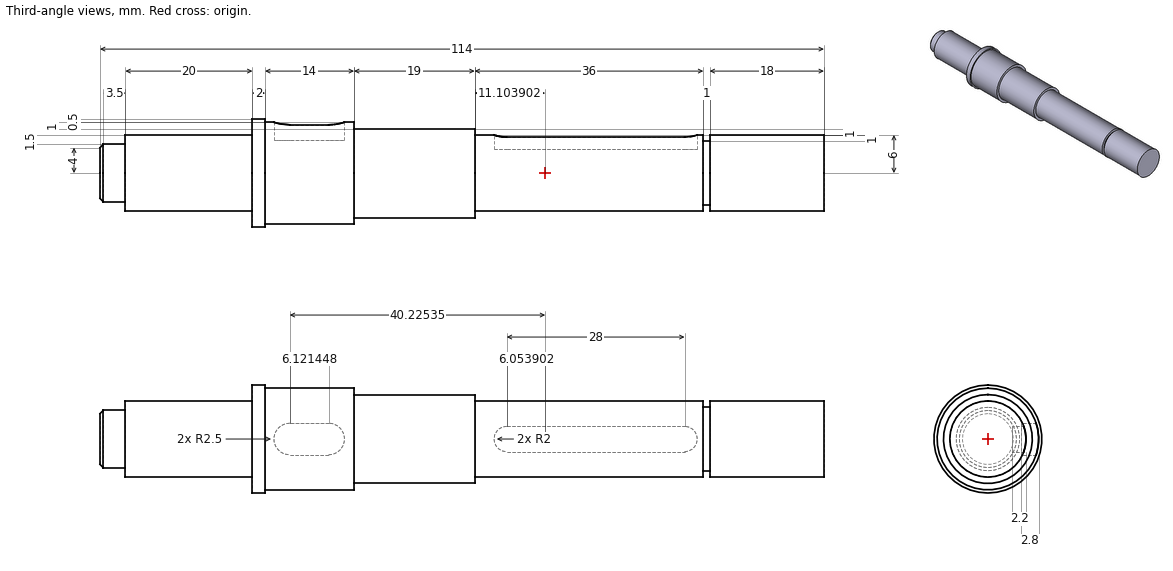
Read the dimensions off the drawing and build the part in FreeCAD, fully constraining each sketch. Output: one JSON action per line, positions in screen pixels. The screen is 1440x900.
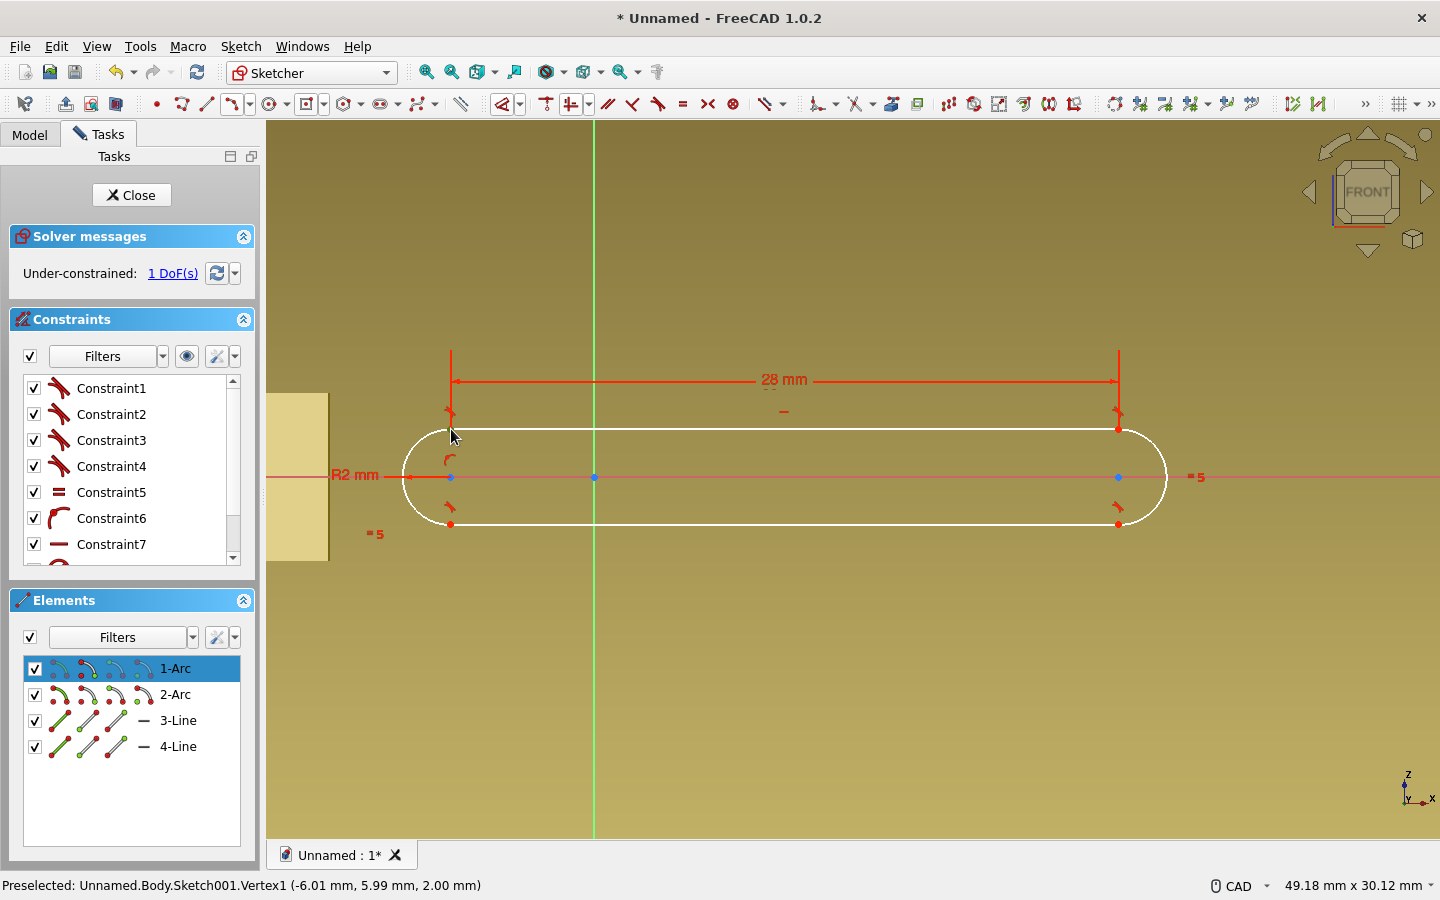
{"action": "left_click", "coordinate": [520, 104]}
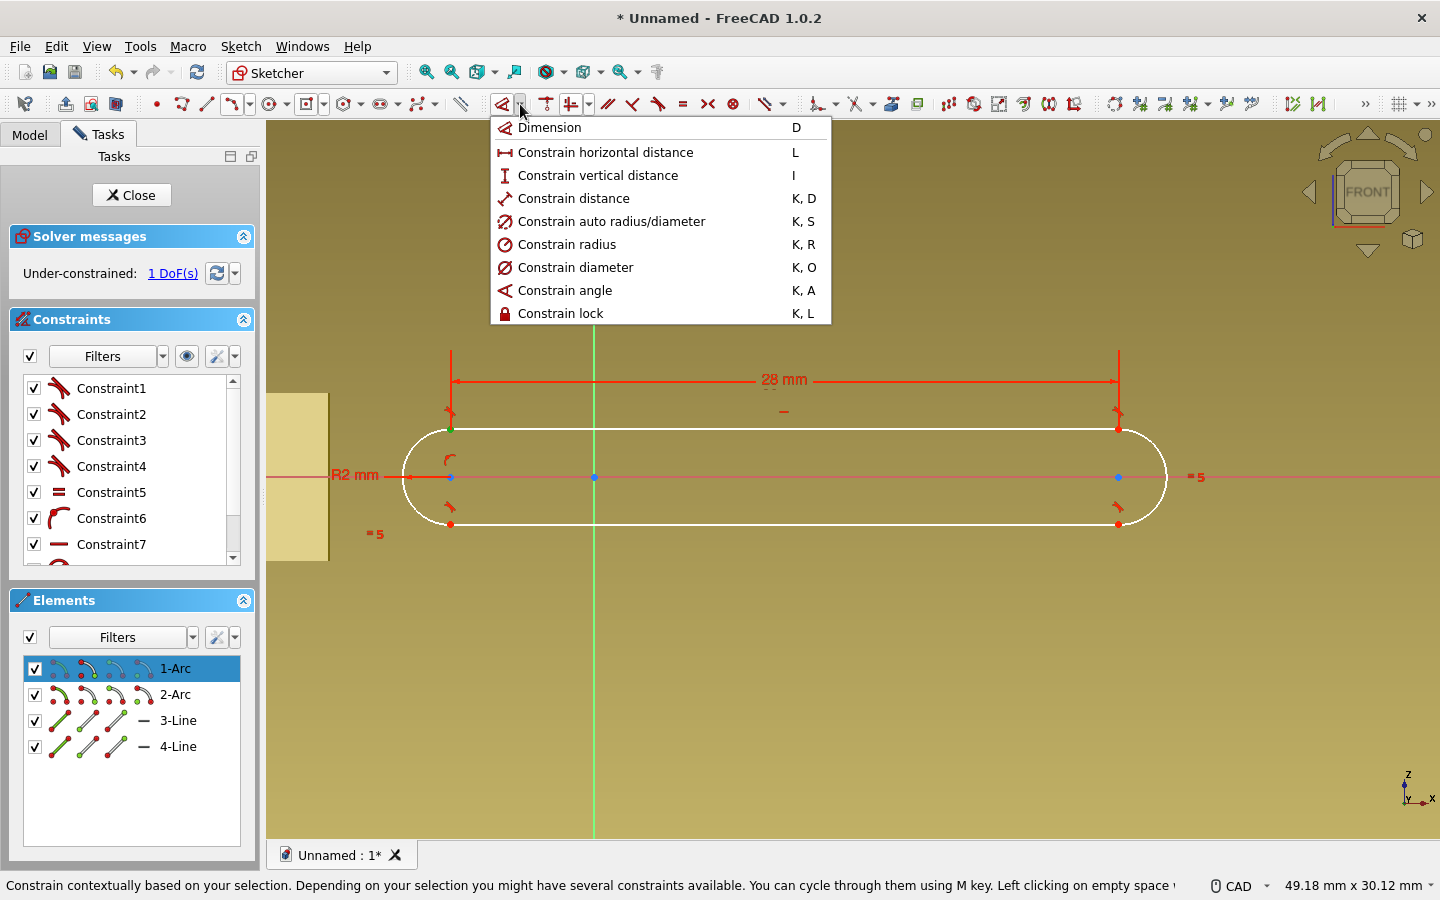
{"action": "left_click", "coordinate": [661, 152]}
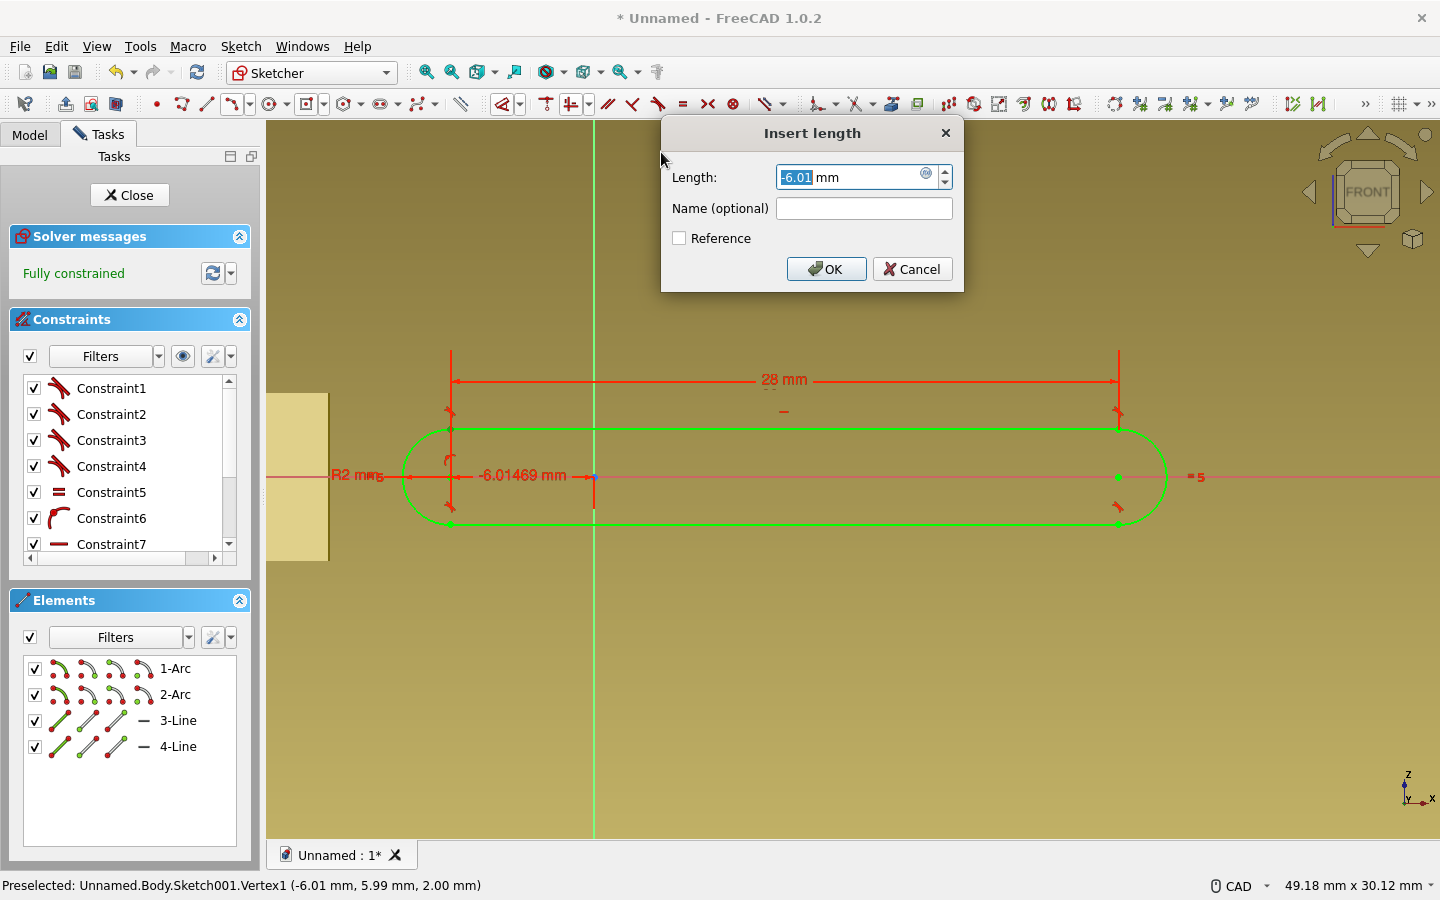
{"action": "type", "text": "-6.053902"}
{"action": "key", "text": "Return"}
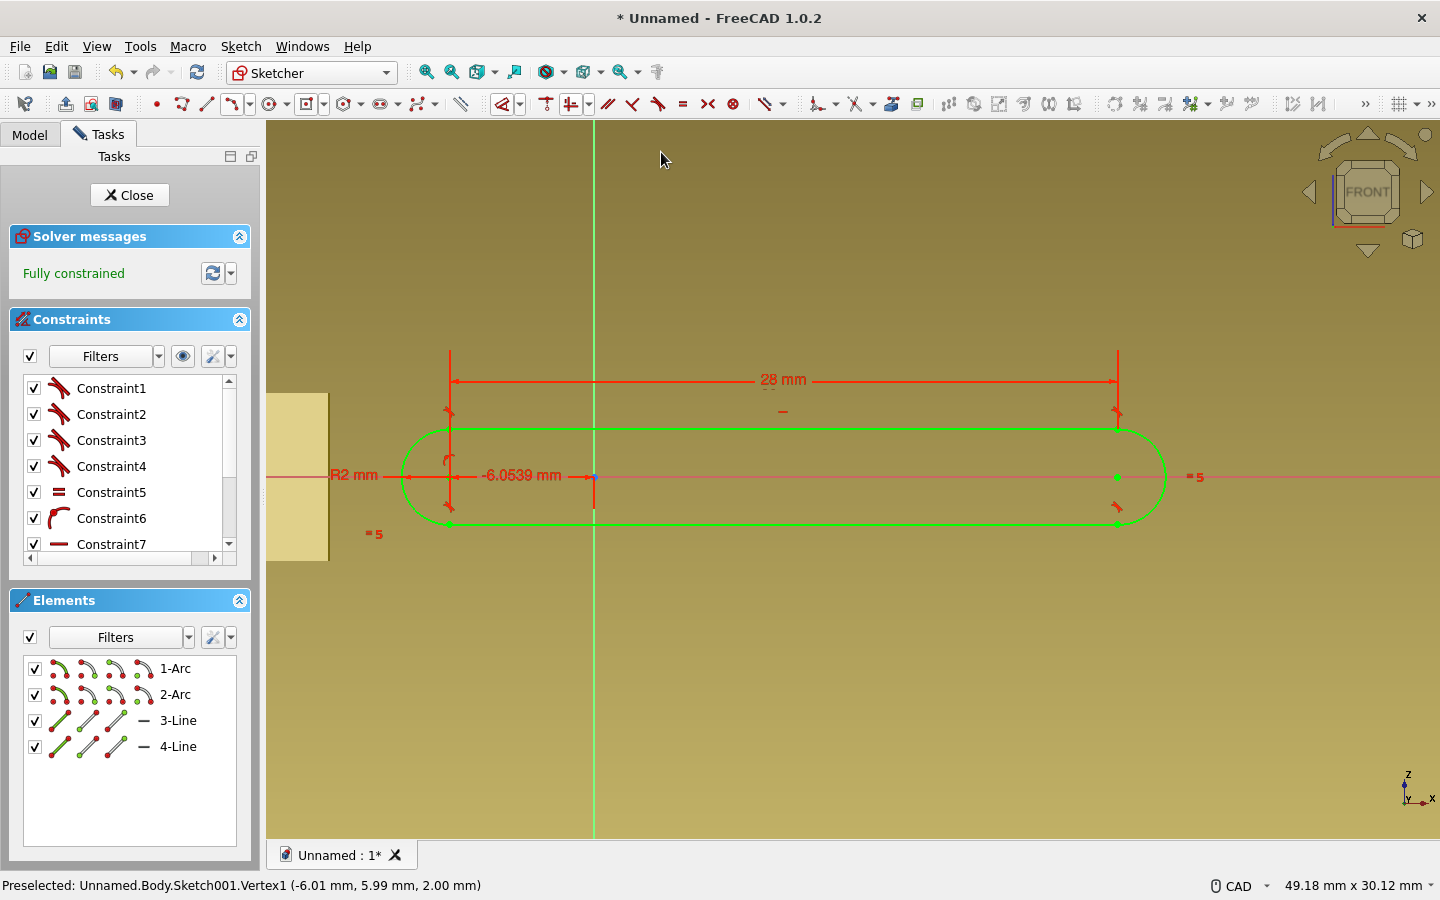
{"action": "left_click", "coordinate": [130, 195]}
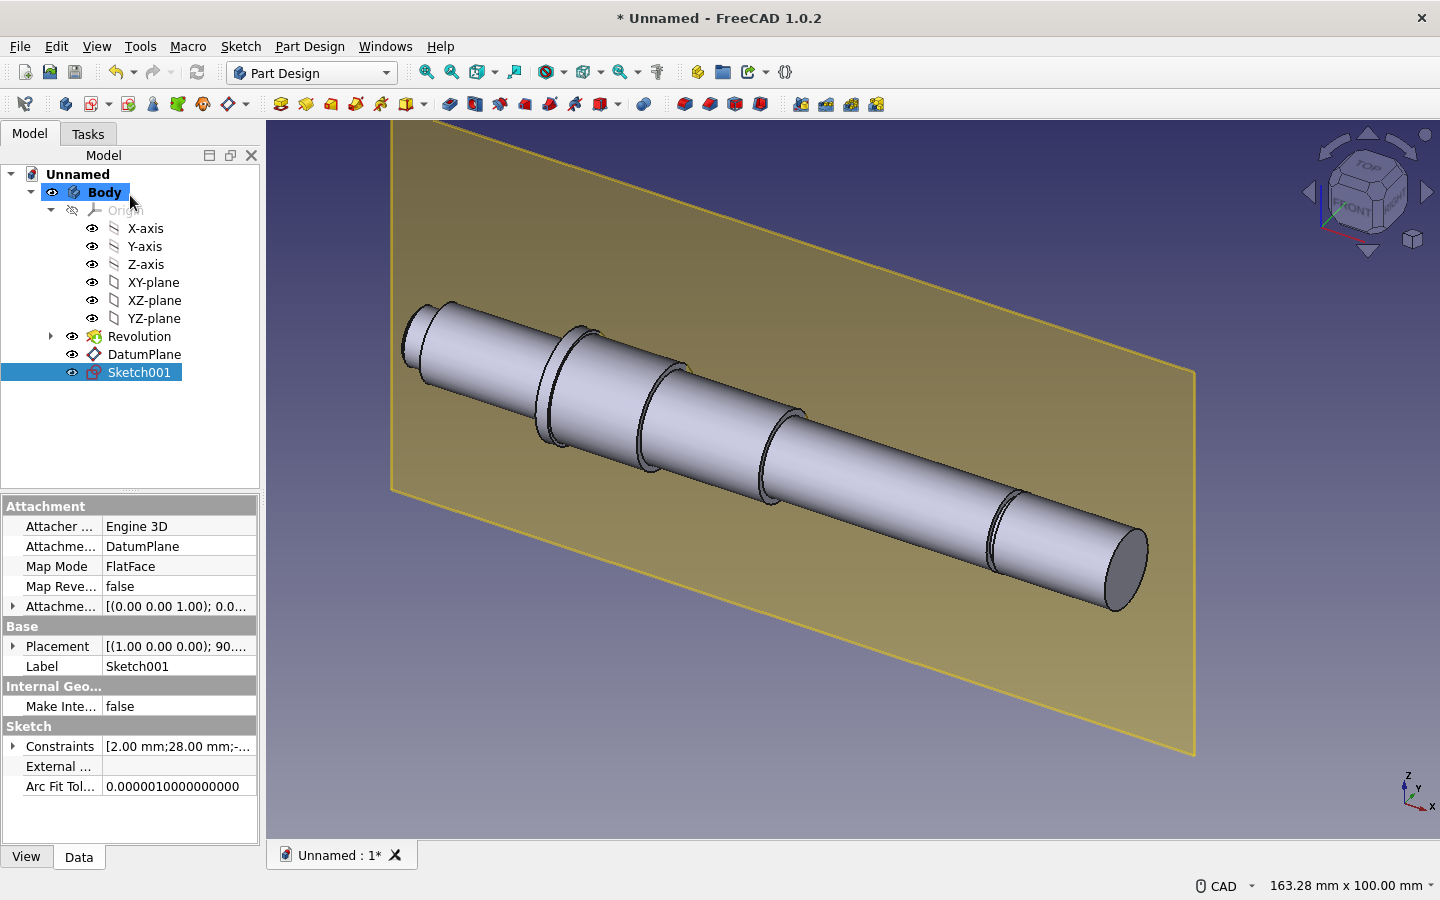
{"action": "left_click", "coordinate": [450, 104]}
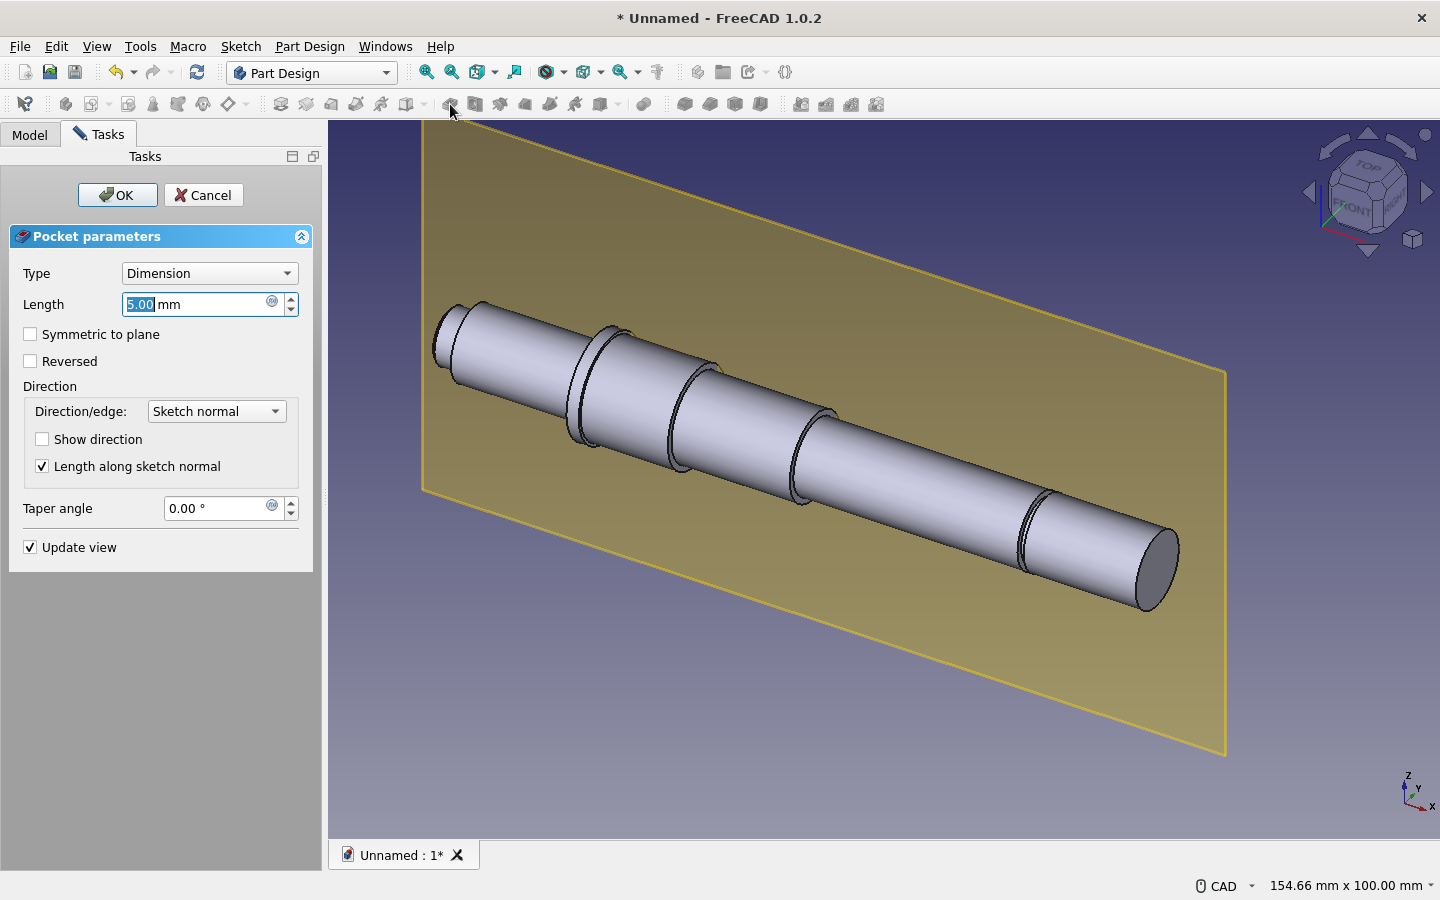
{"action": "type", "text": "2.2"}
{"action": "key", "text": "Tab"}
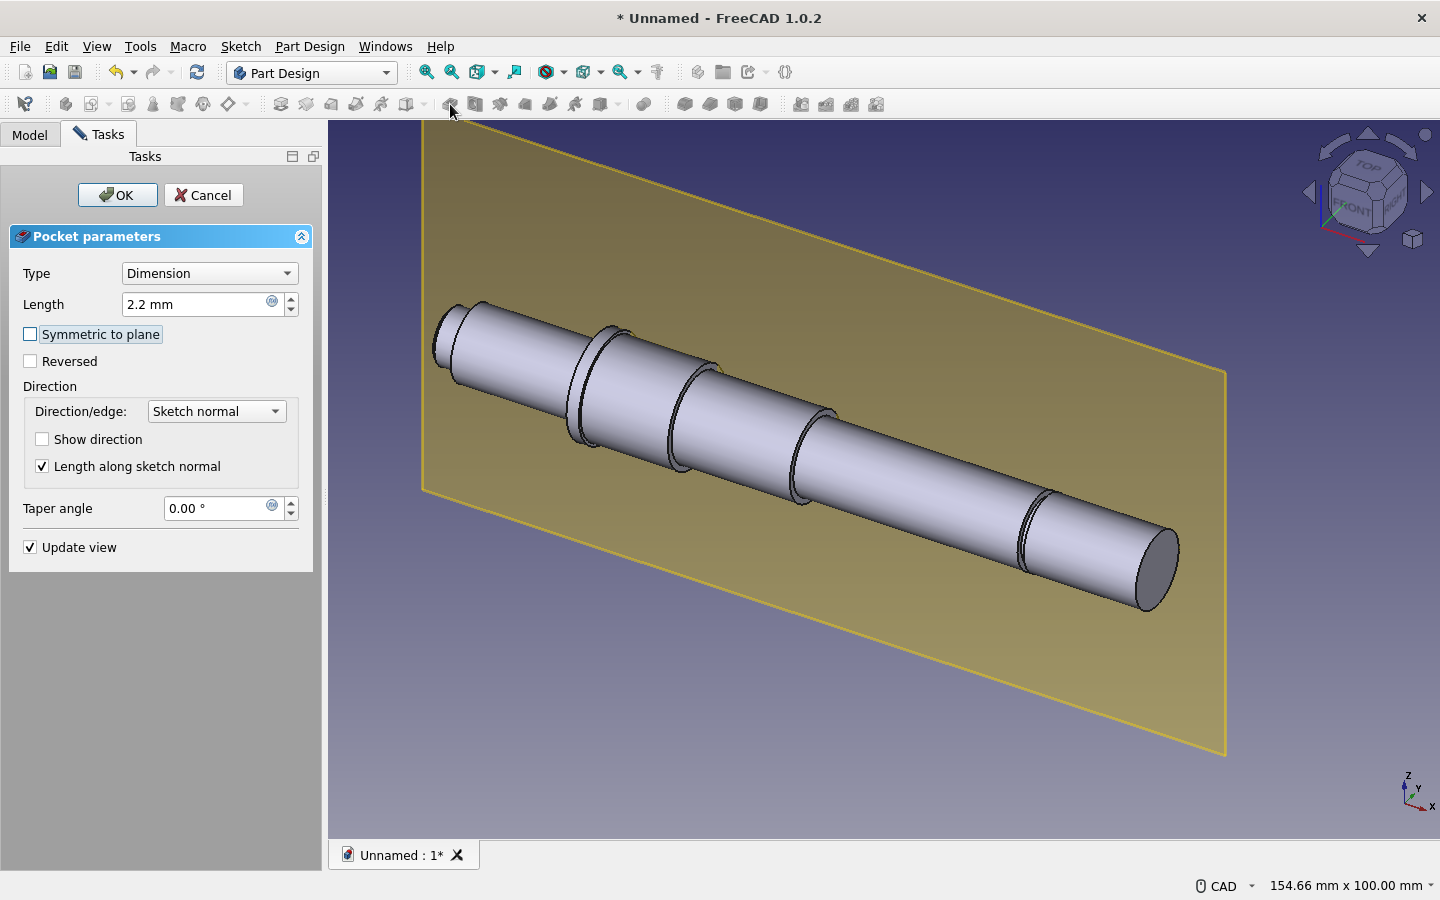
{"action": "left_click", "coordinate": [31, 361]}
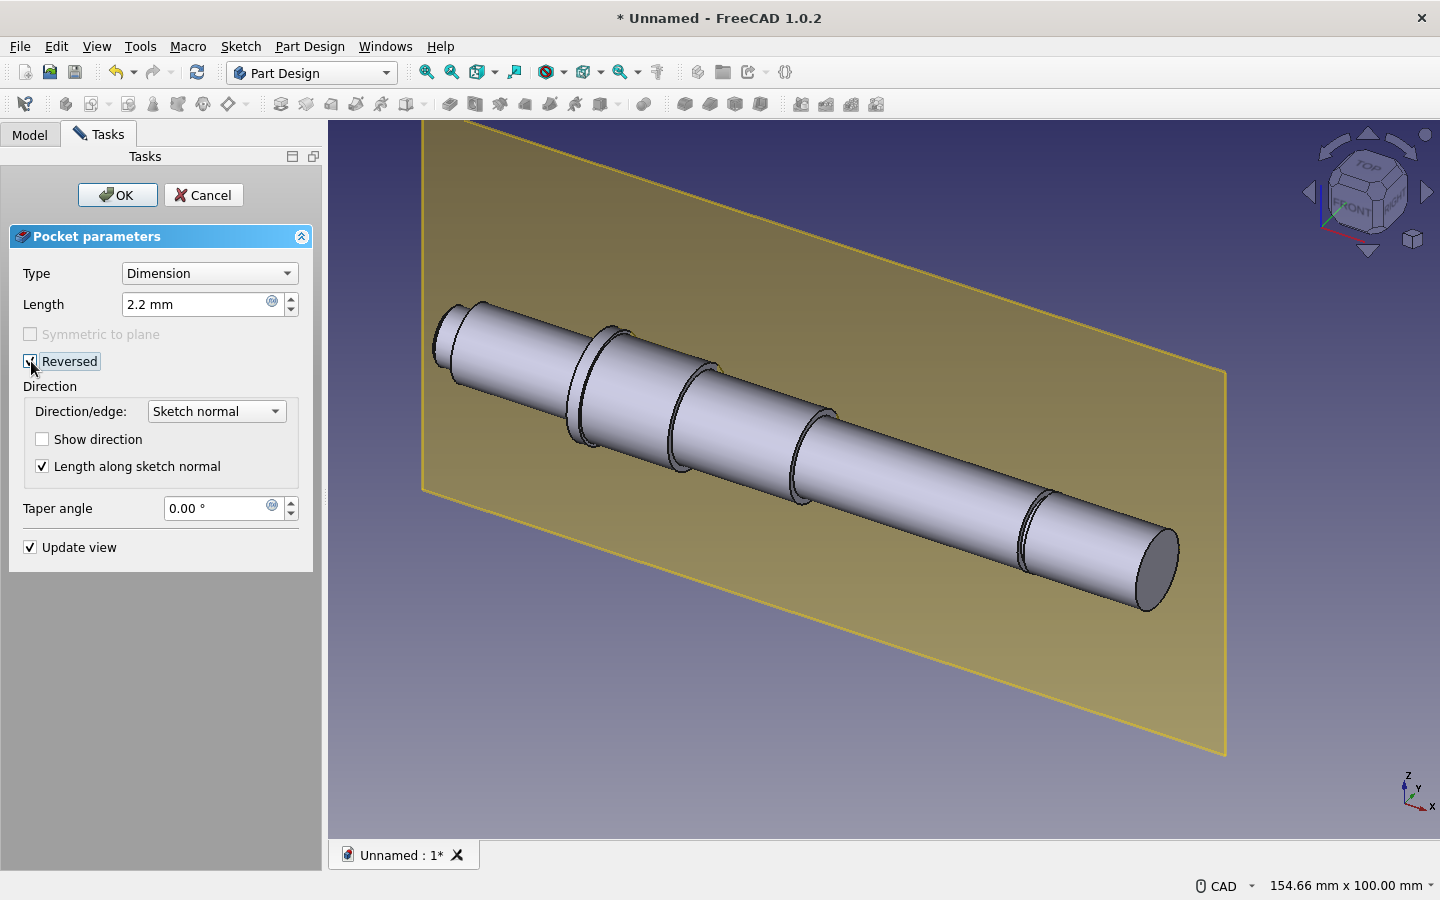
{"action": "left_click", "coordinate": [118, 195]}